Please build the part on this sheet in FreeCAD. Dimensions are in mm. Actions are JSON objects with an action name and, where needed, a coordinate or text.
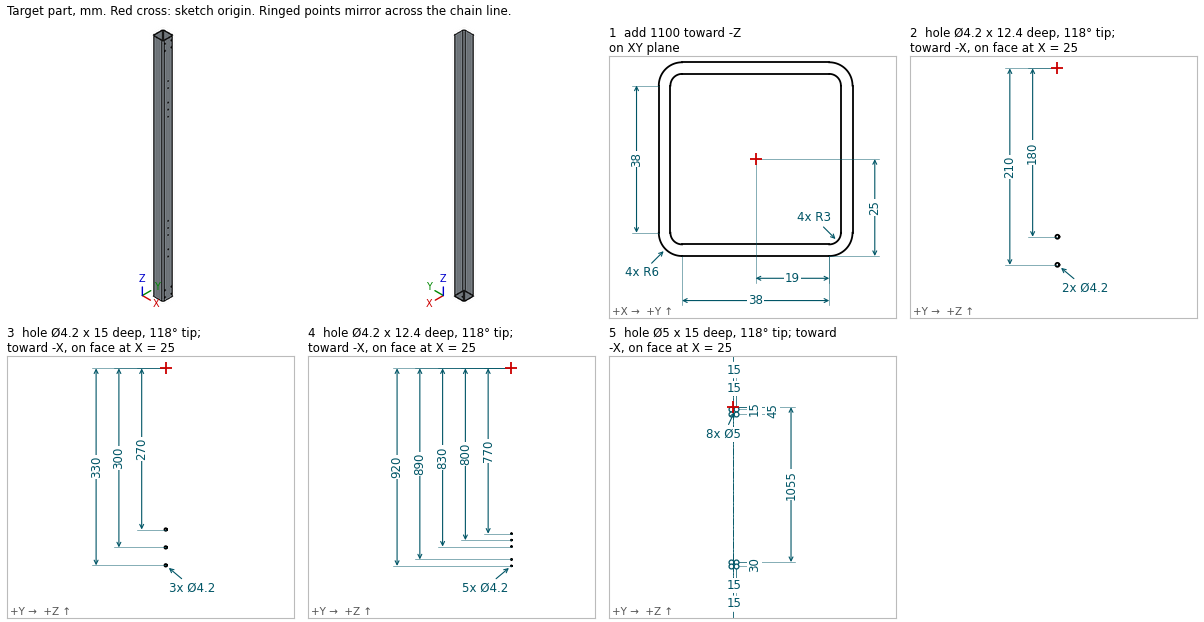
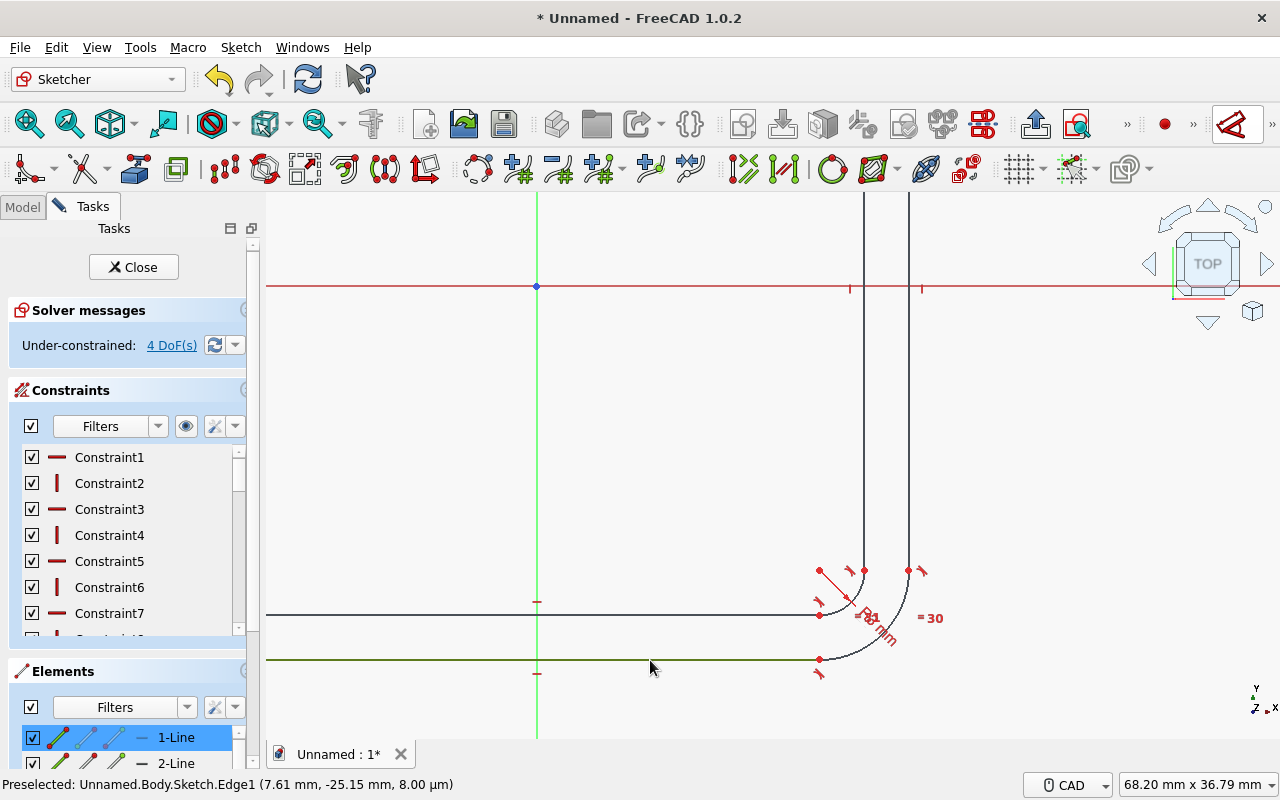
{"action": "left_click", "coordinate": [1258, 124]}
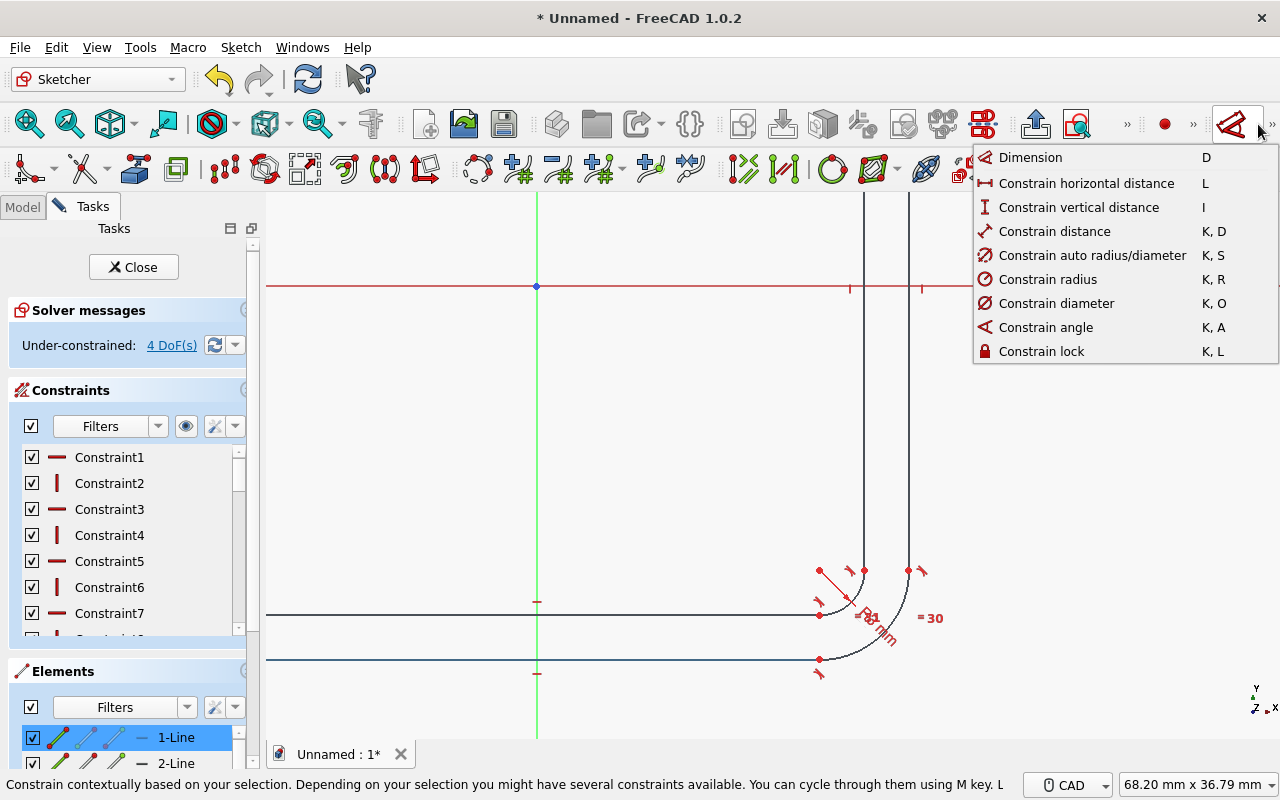
{"action": "left_click", "coordinate": [1126, 183]}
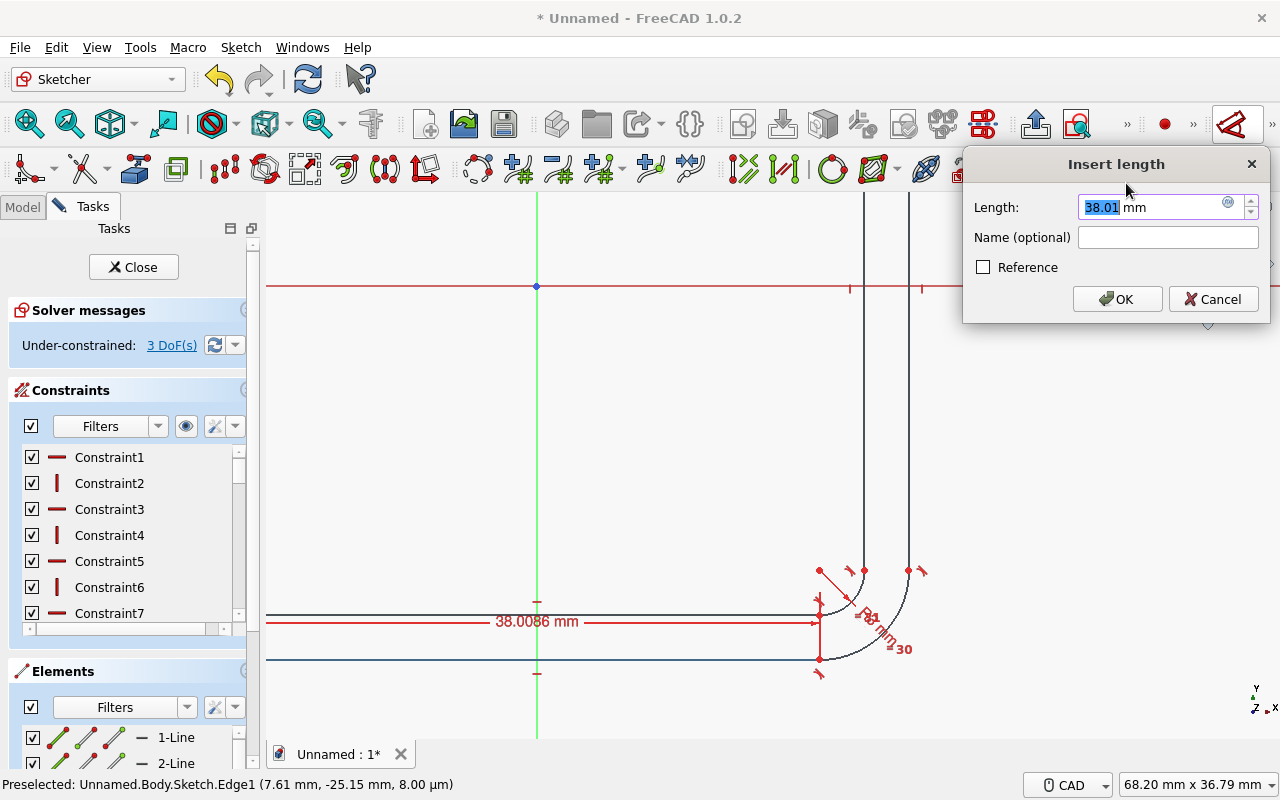
{"action": "type", "text": "38"}
{"action": "key", "text": "Return"}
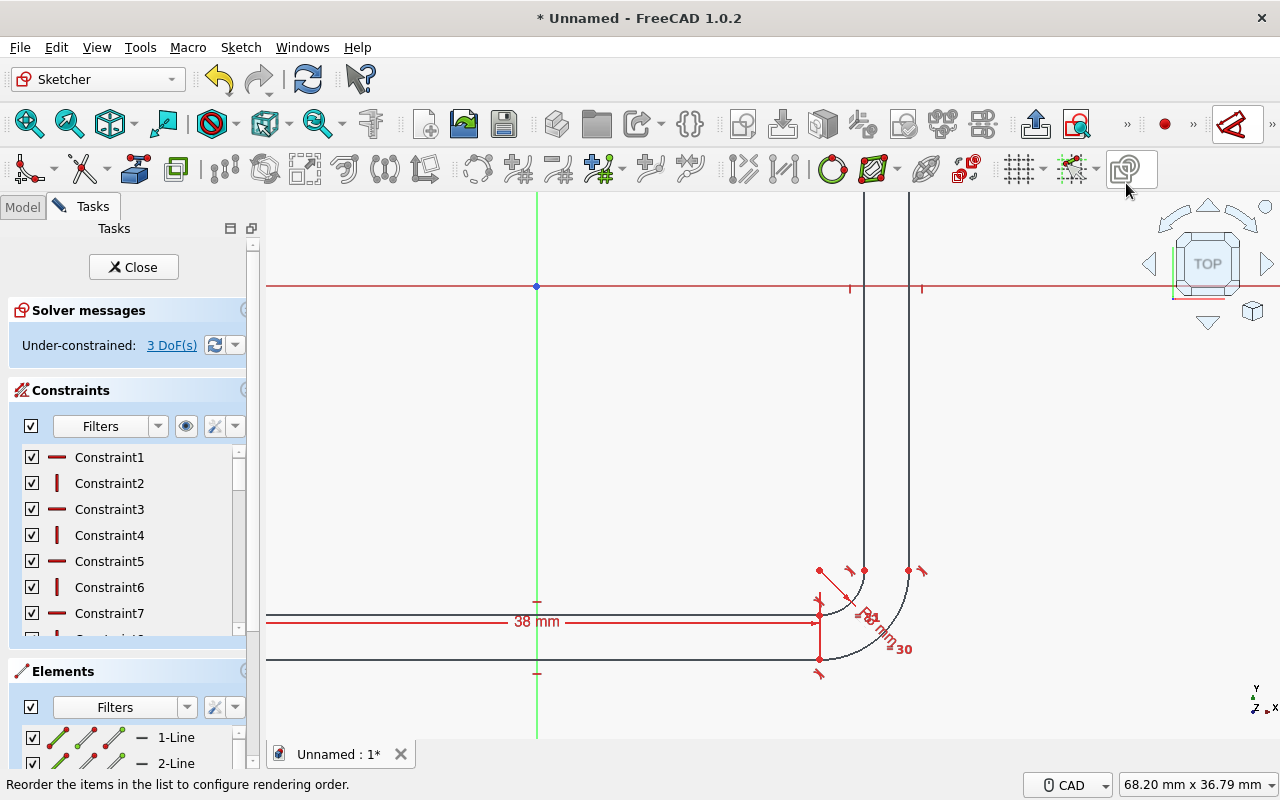
{"action": "scroll", "coordinate": [841, 612], "scroll_direction": "down", "scroll_amount": 4}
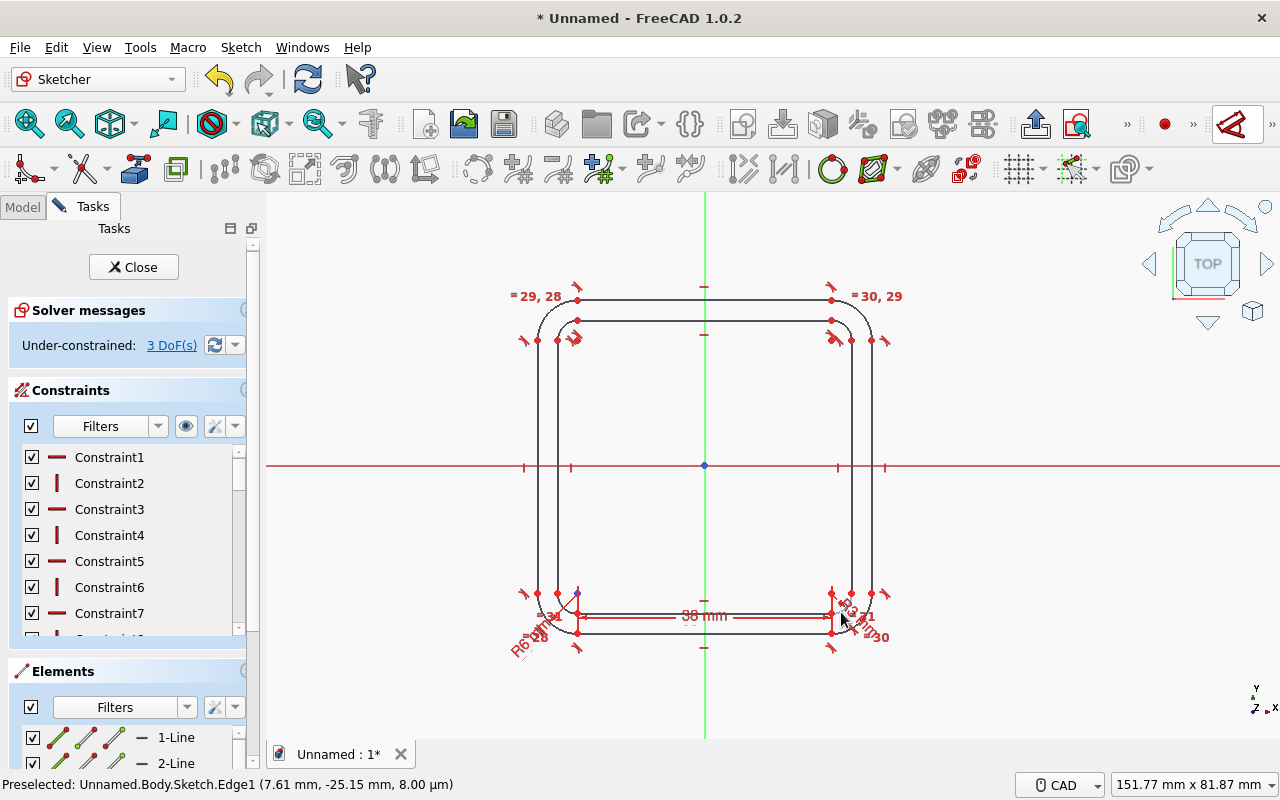
{"action": "left_click", "coordinate": [538, 518]}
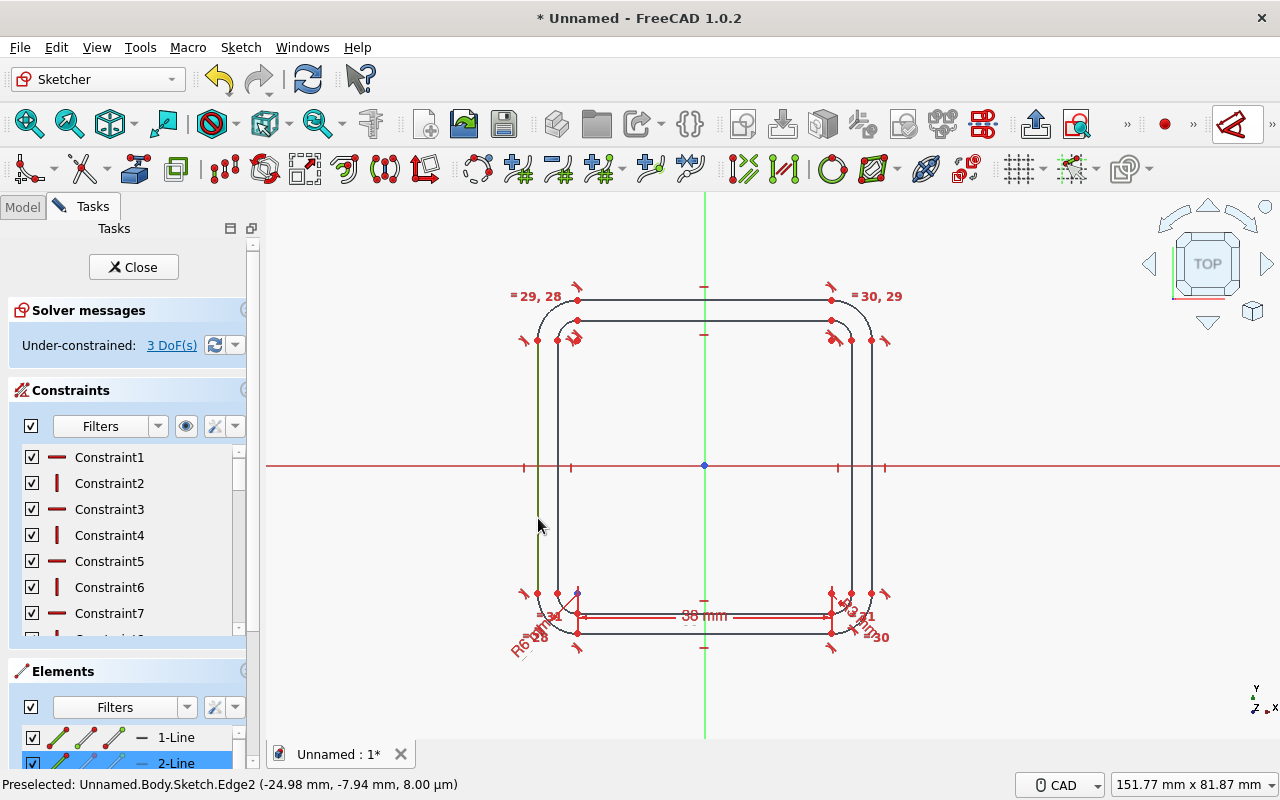
{"action": "left_click", "coordinate": [1258, 124]}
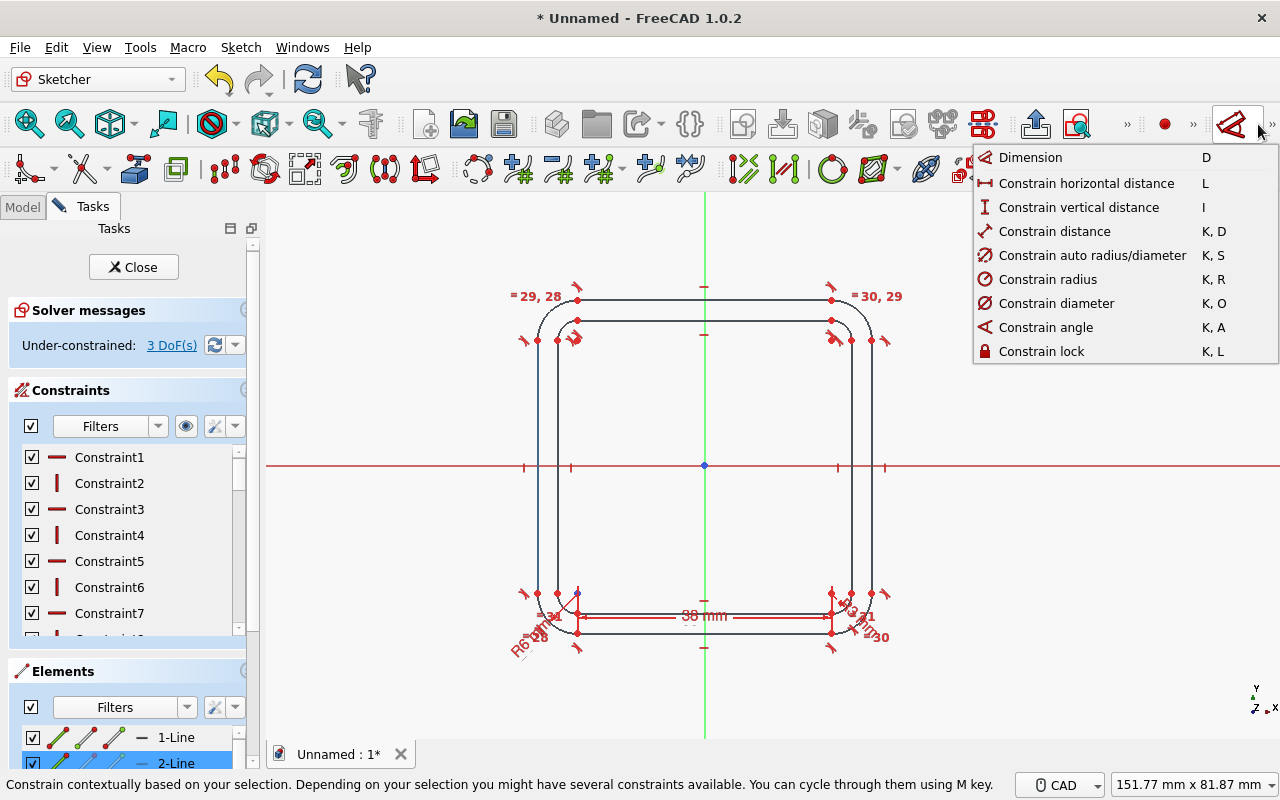
{"action": "left_click", "coordinate": [1126, 207]}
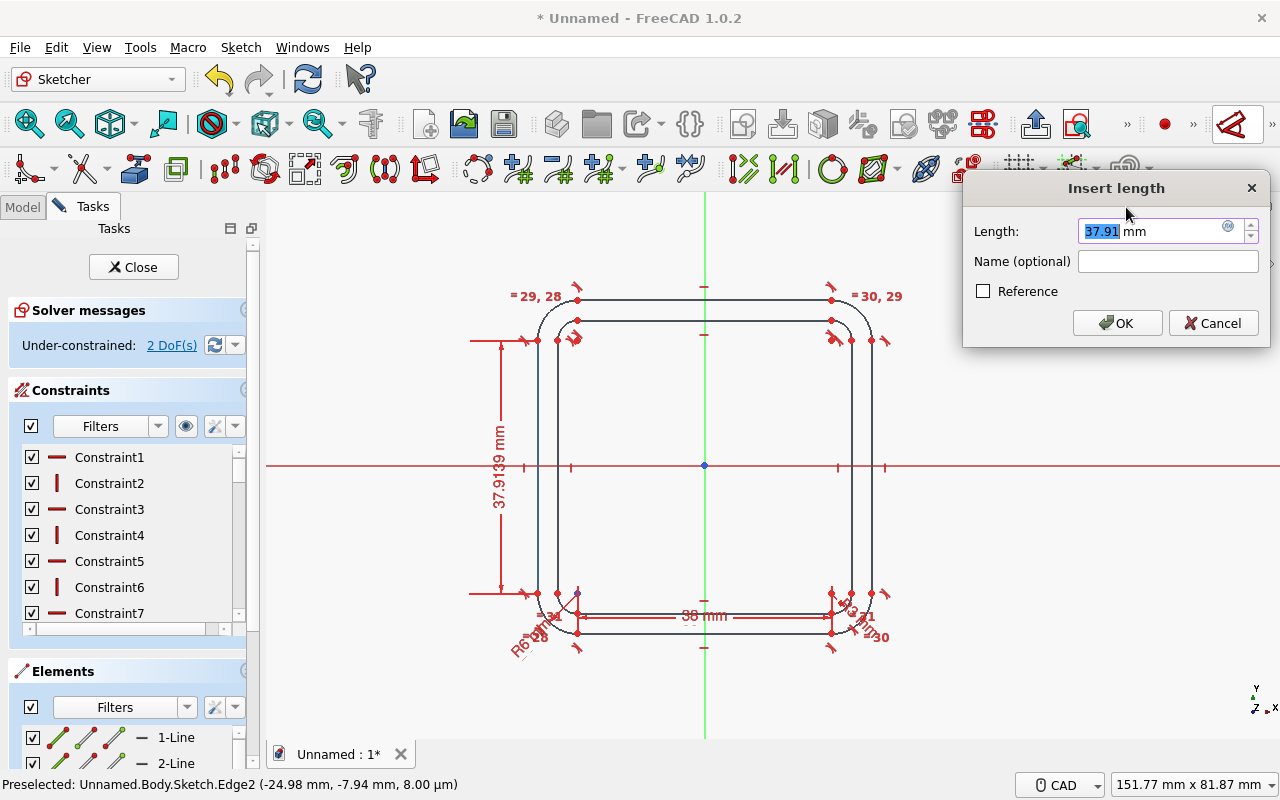
{"action": "type", "text": "38"}
{"action": "key", "text": "Return"}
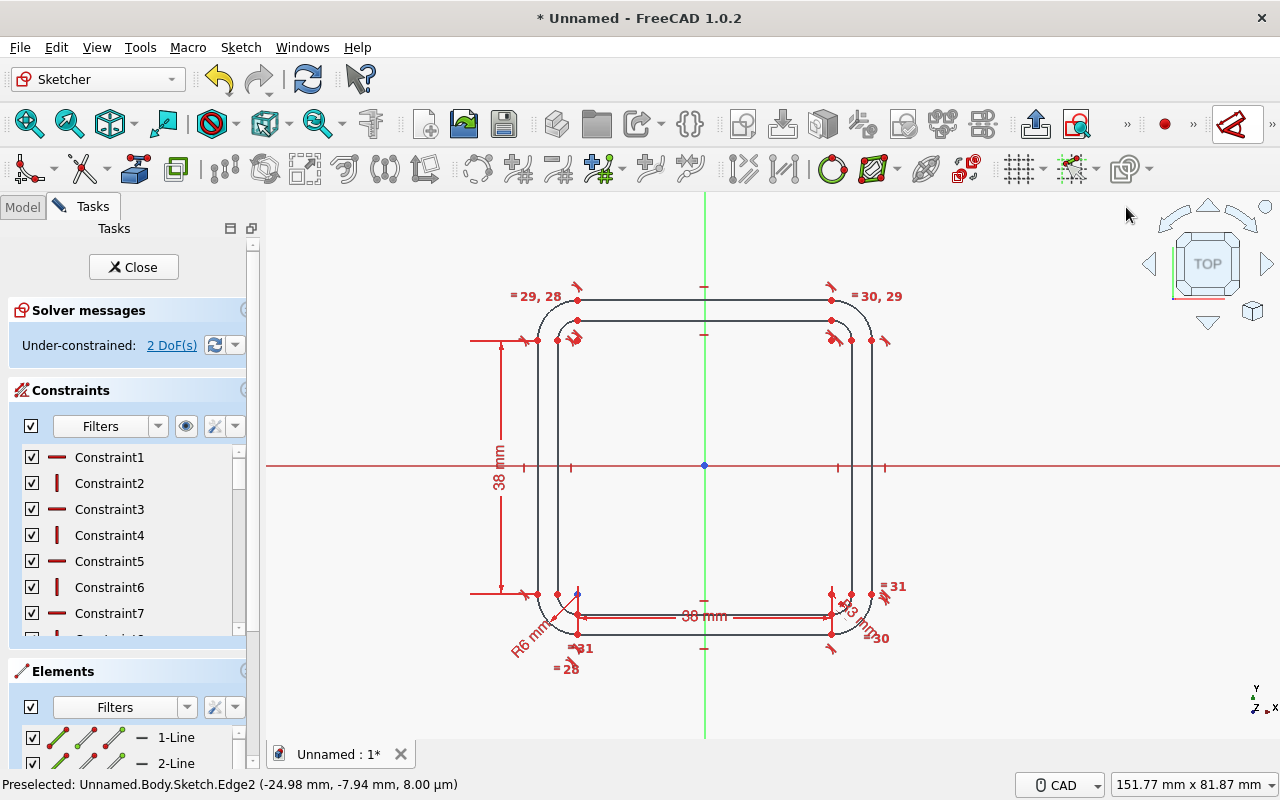
{"action": "left_click", "coordinate": [832, 635]}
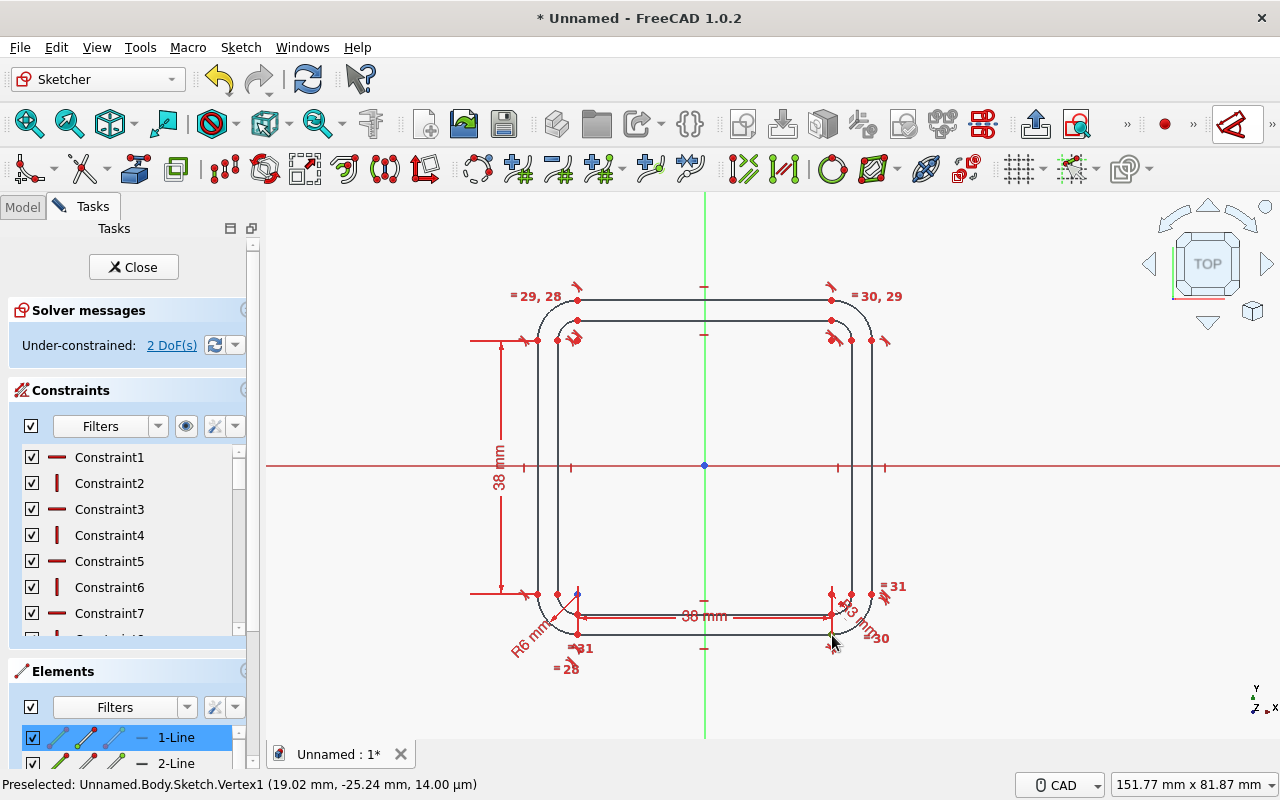
{"action": "key", "text": "l"}